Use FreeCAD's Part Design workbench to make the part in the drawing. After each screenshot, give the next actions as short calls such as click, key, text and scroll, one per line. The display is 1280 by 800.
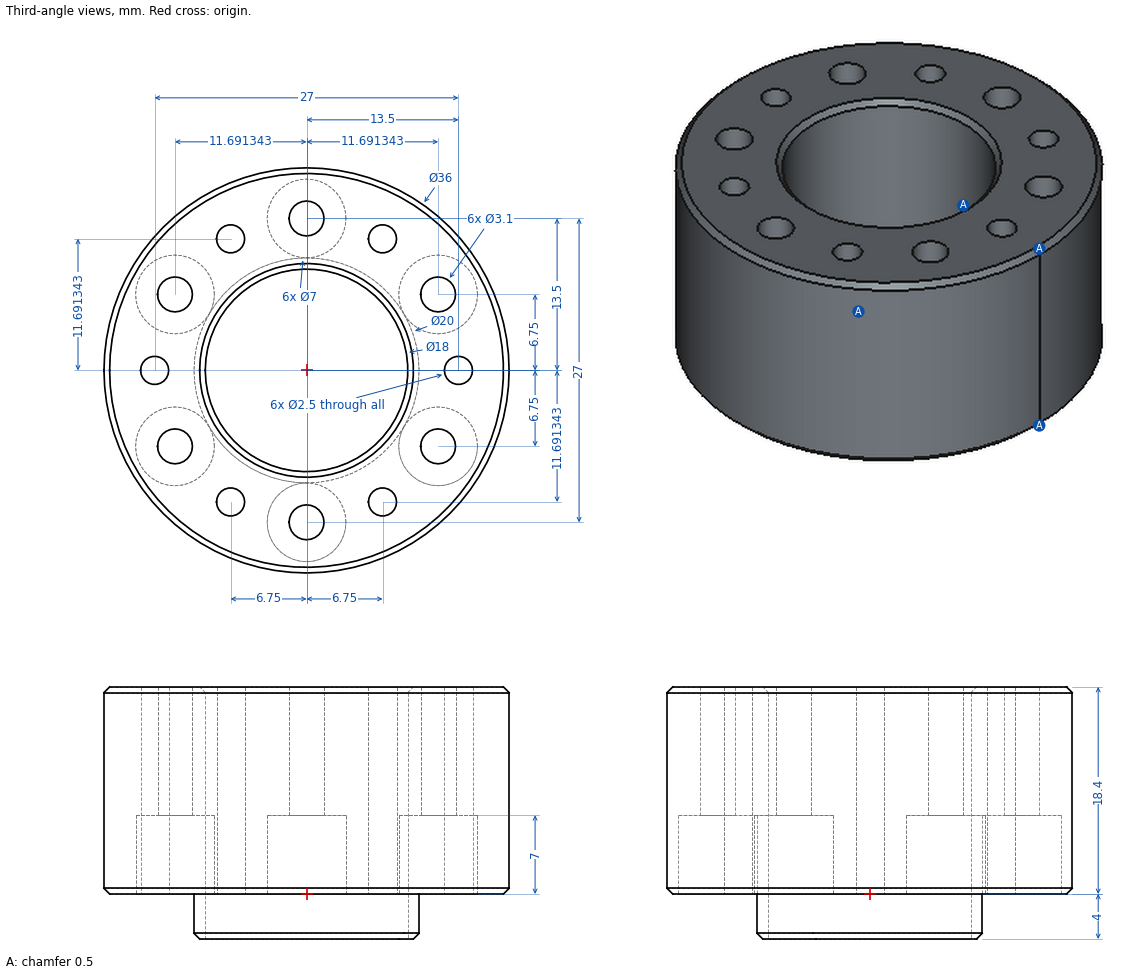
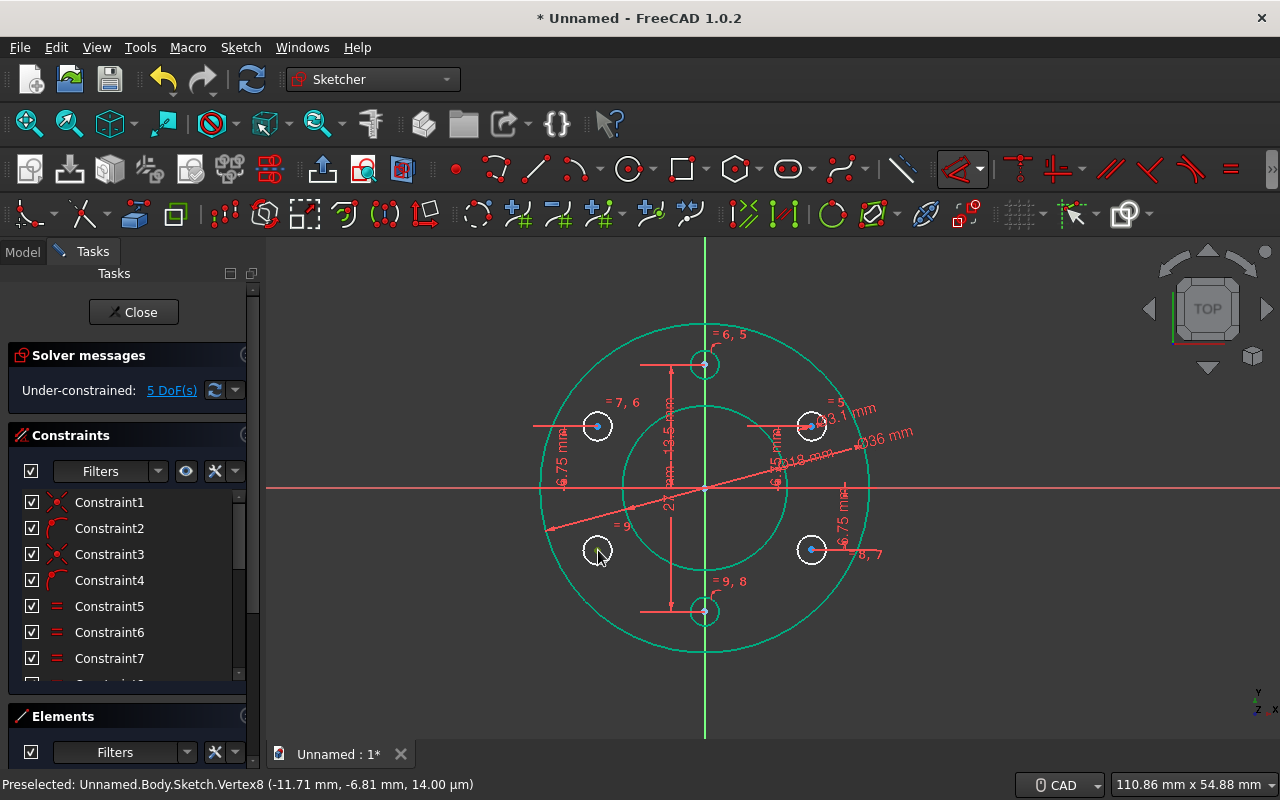
click(982, 170)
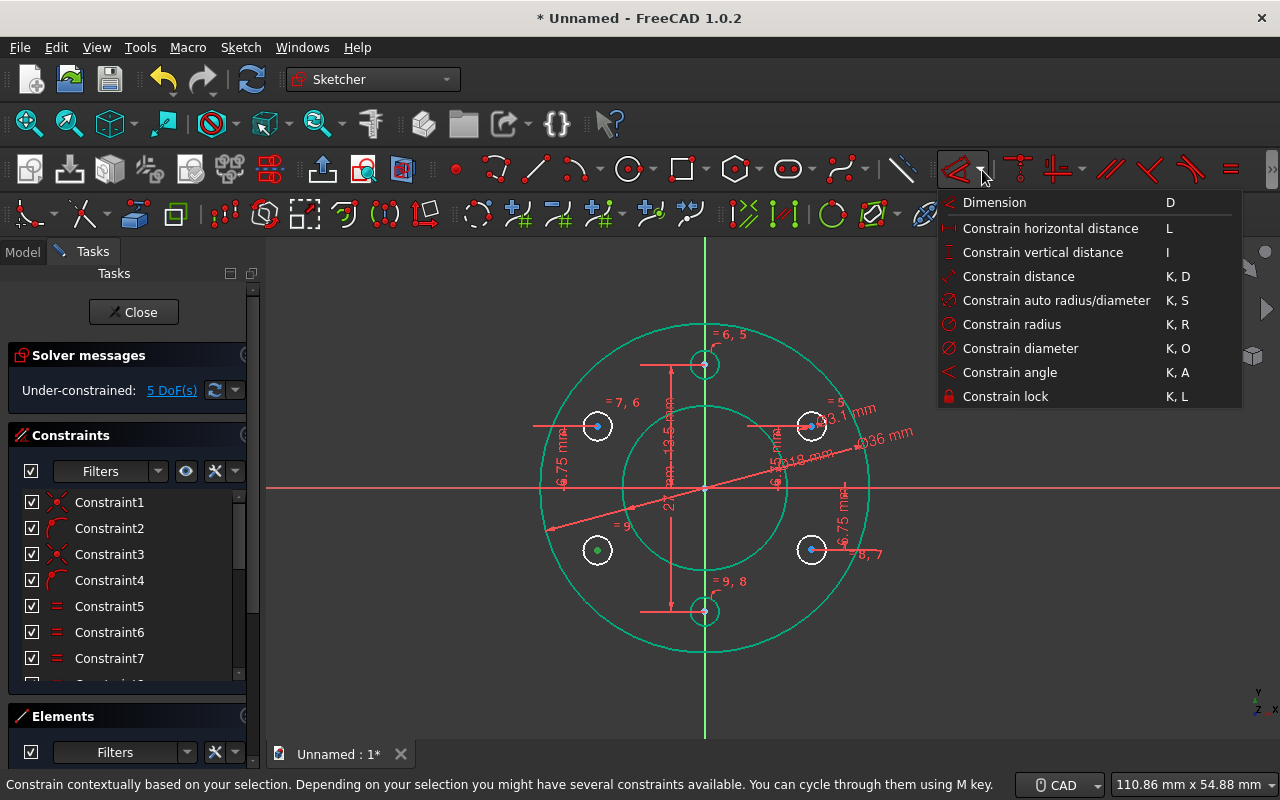
click(1090, 252)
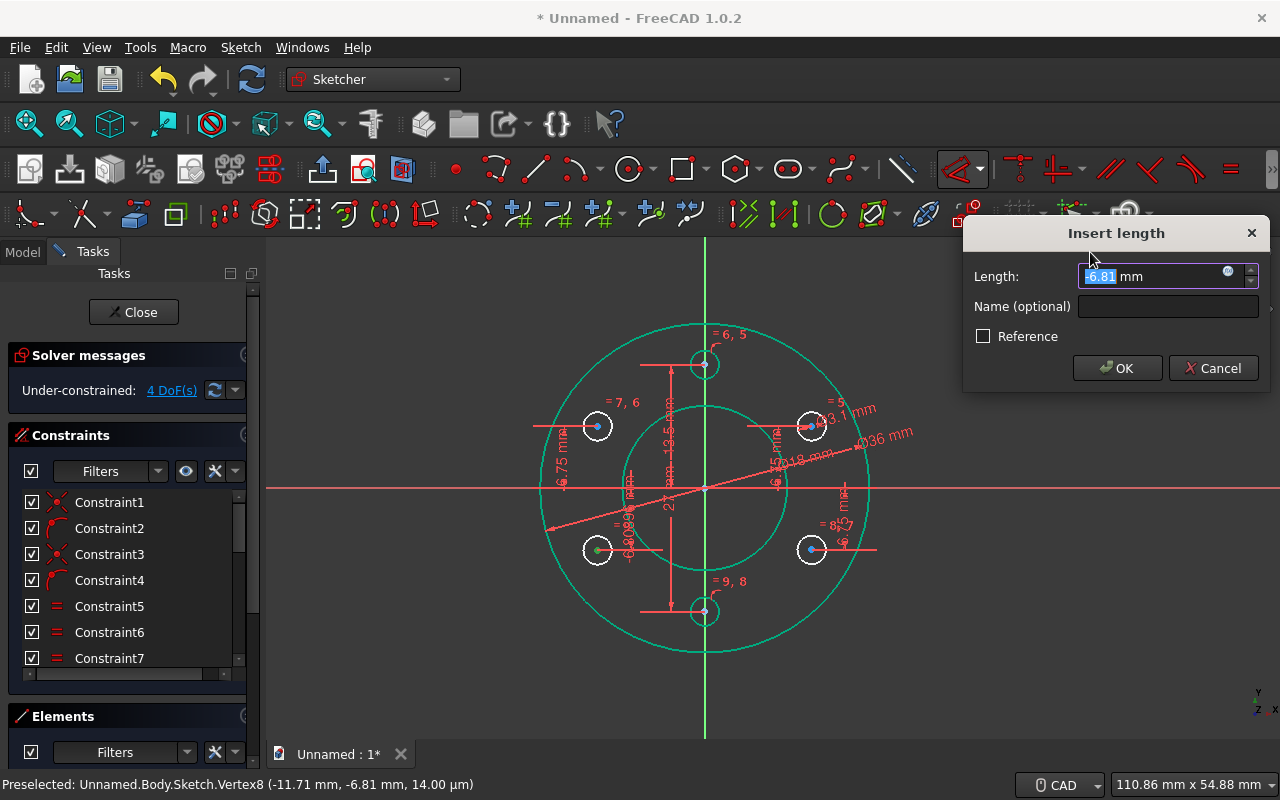
text(-6.75)
key(Return)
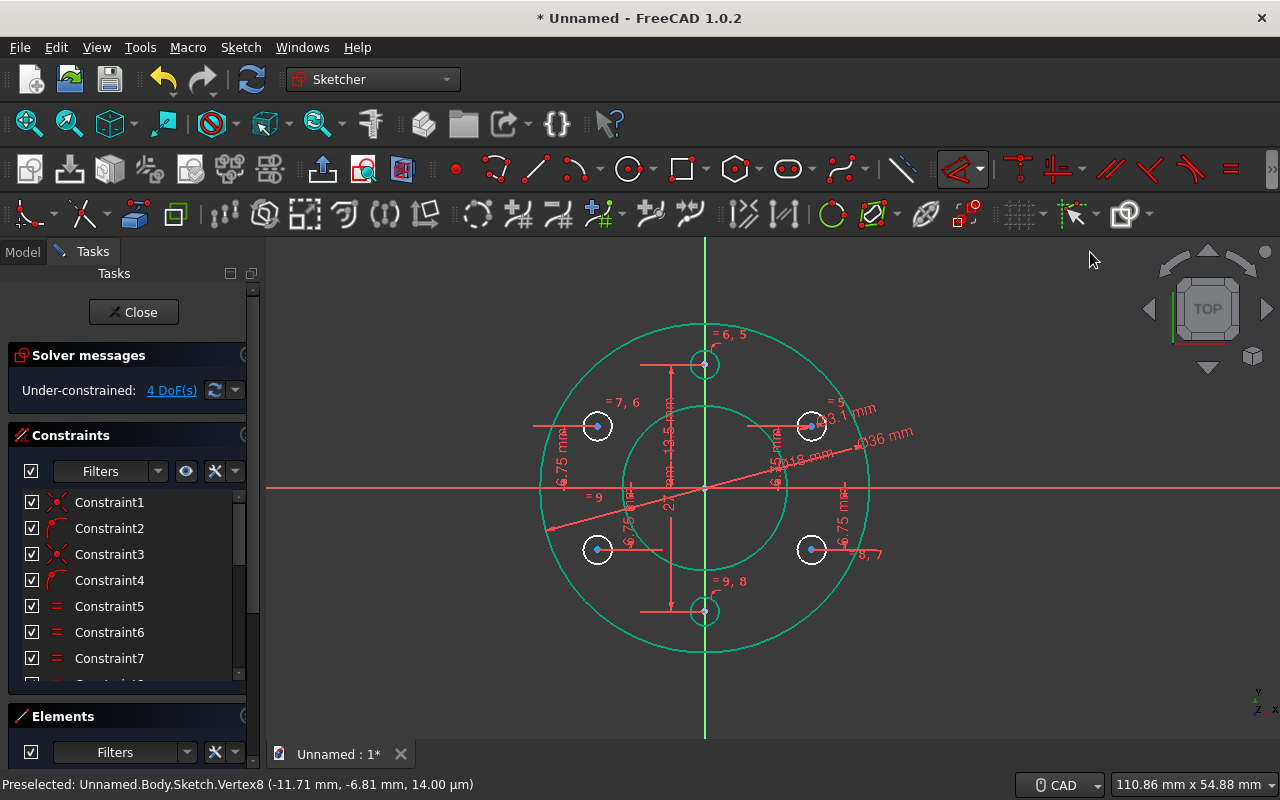
click(812, 426)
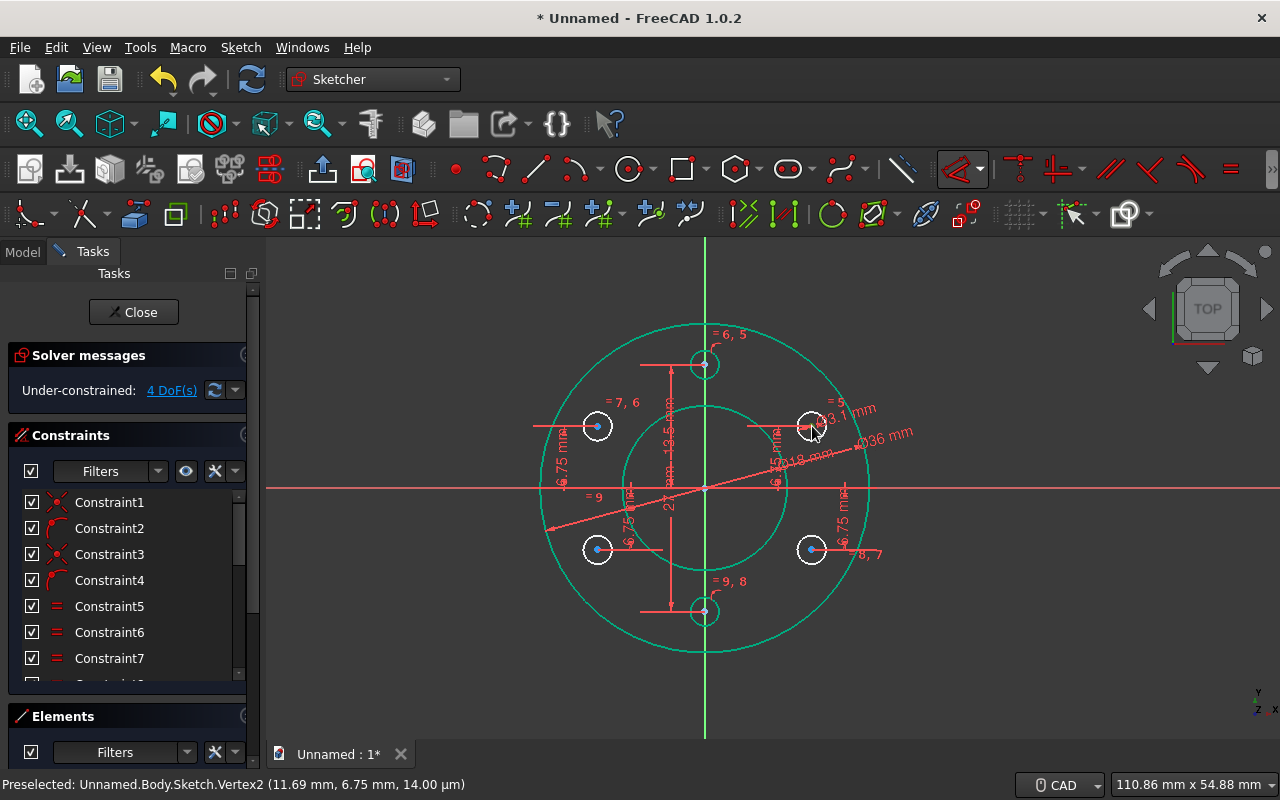
key(l)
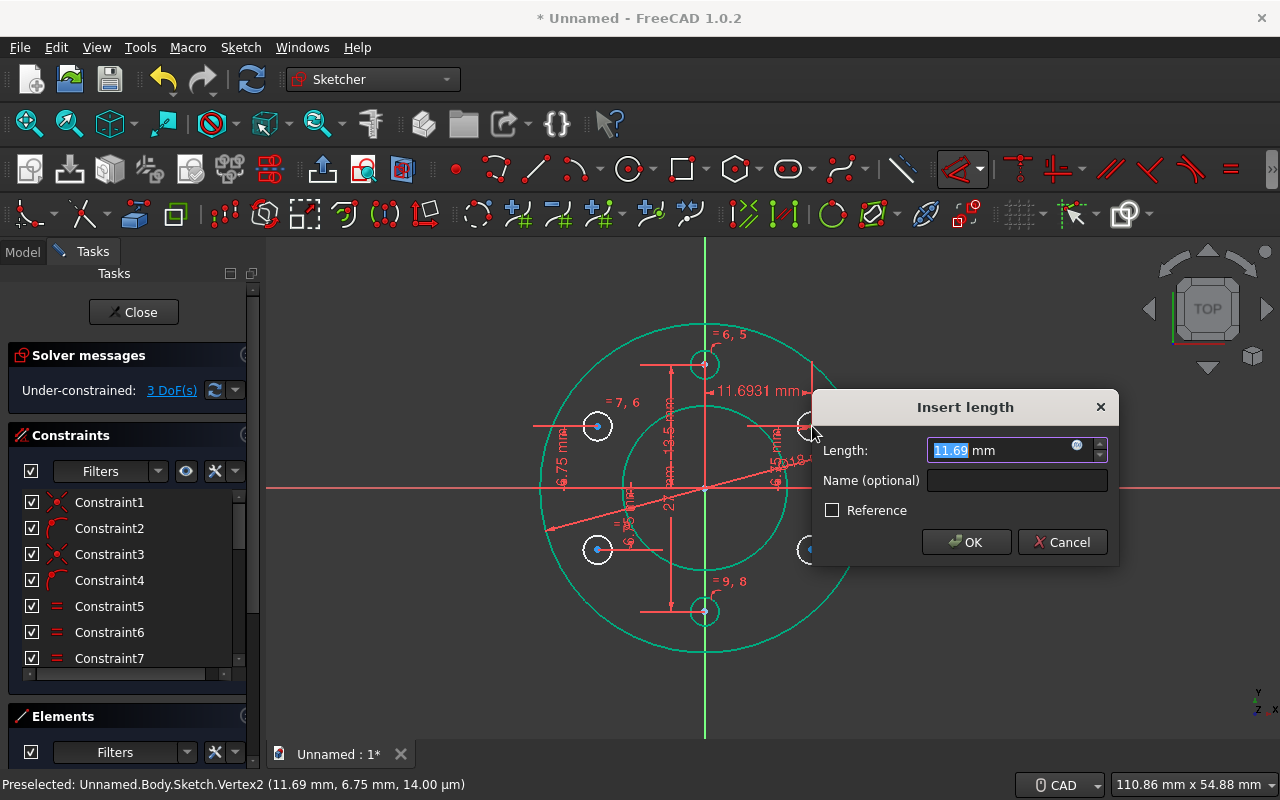
text(11.691343)
key(Return)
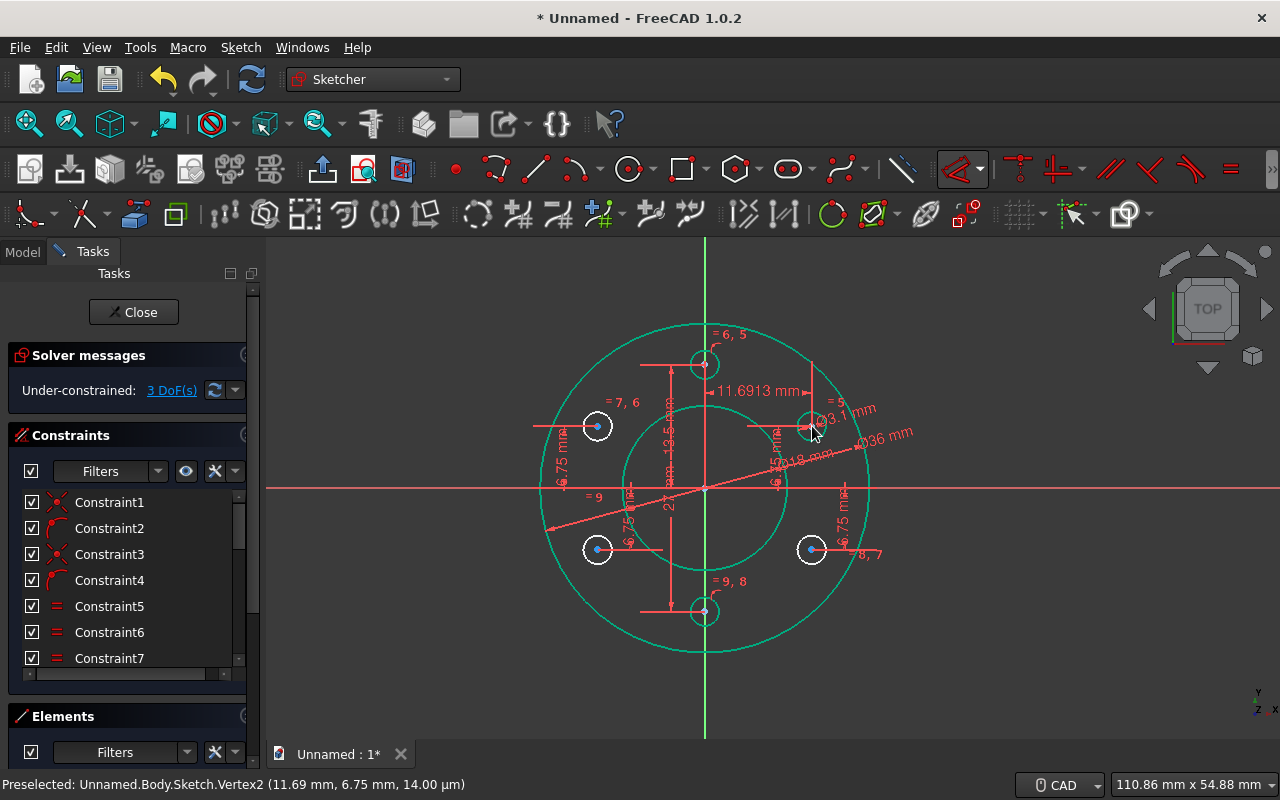
click(598, 426)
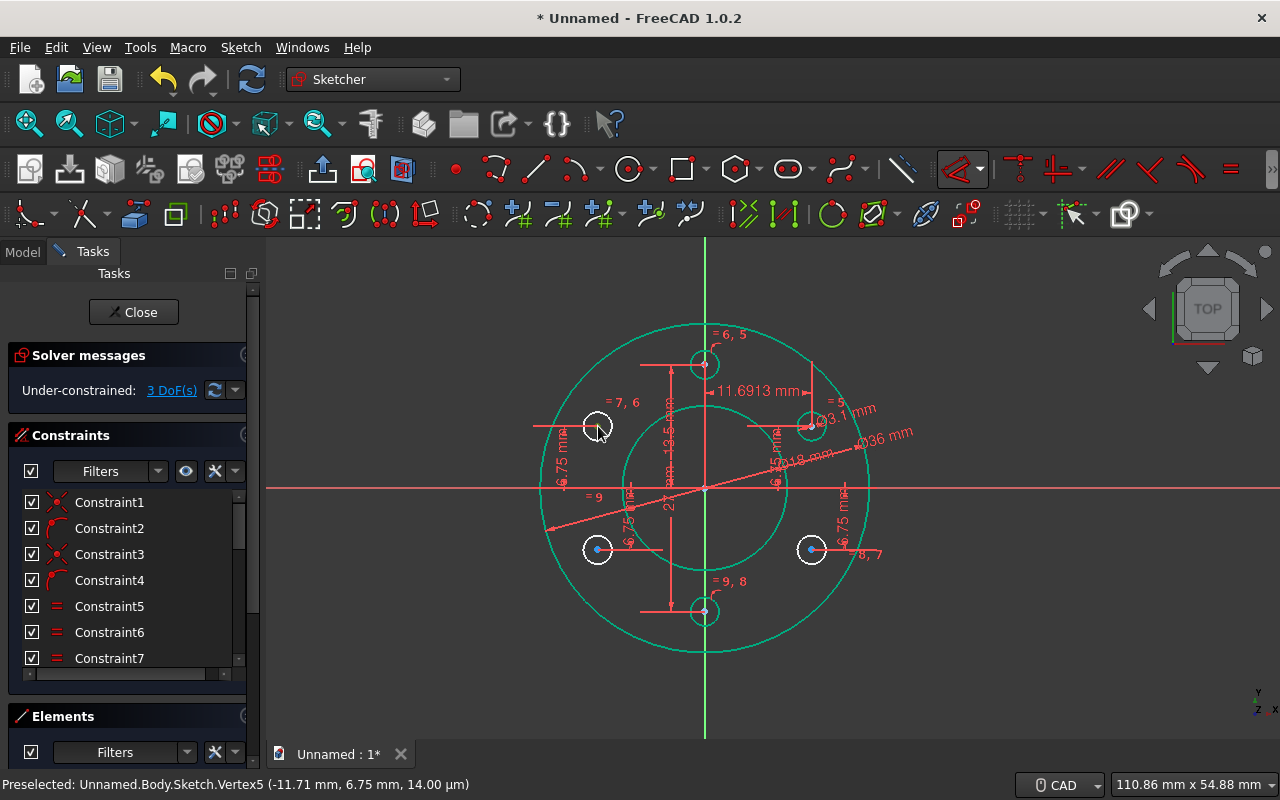
click(982, 170)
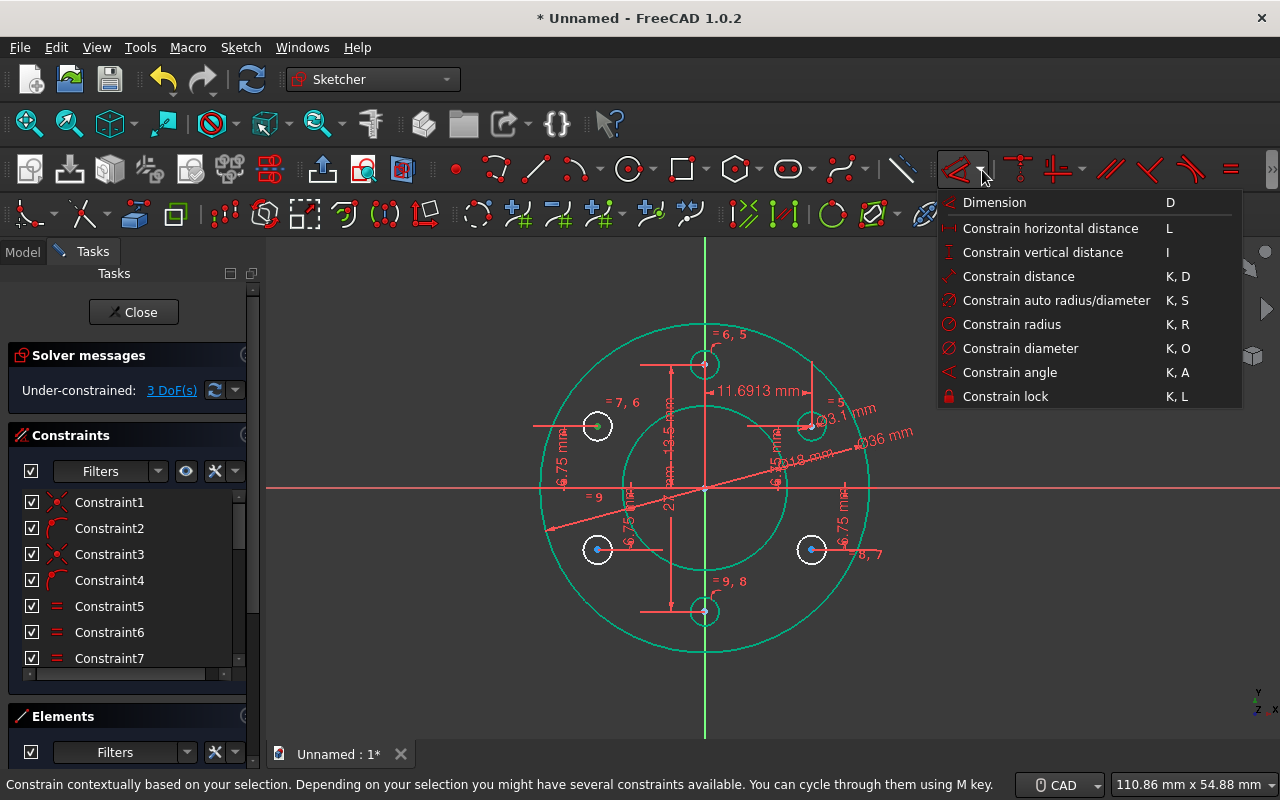
click(1090, 228)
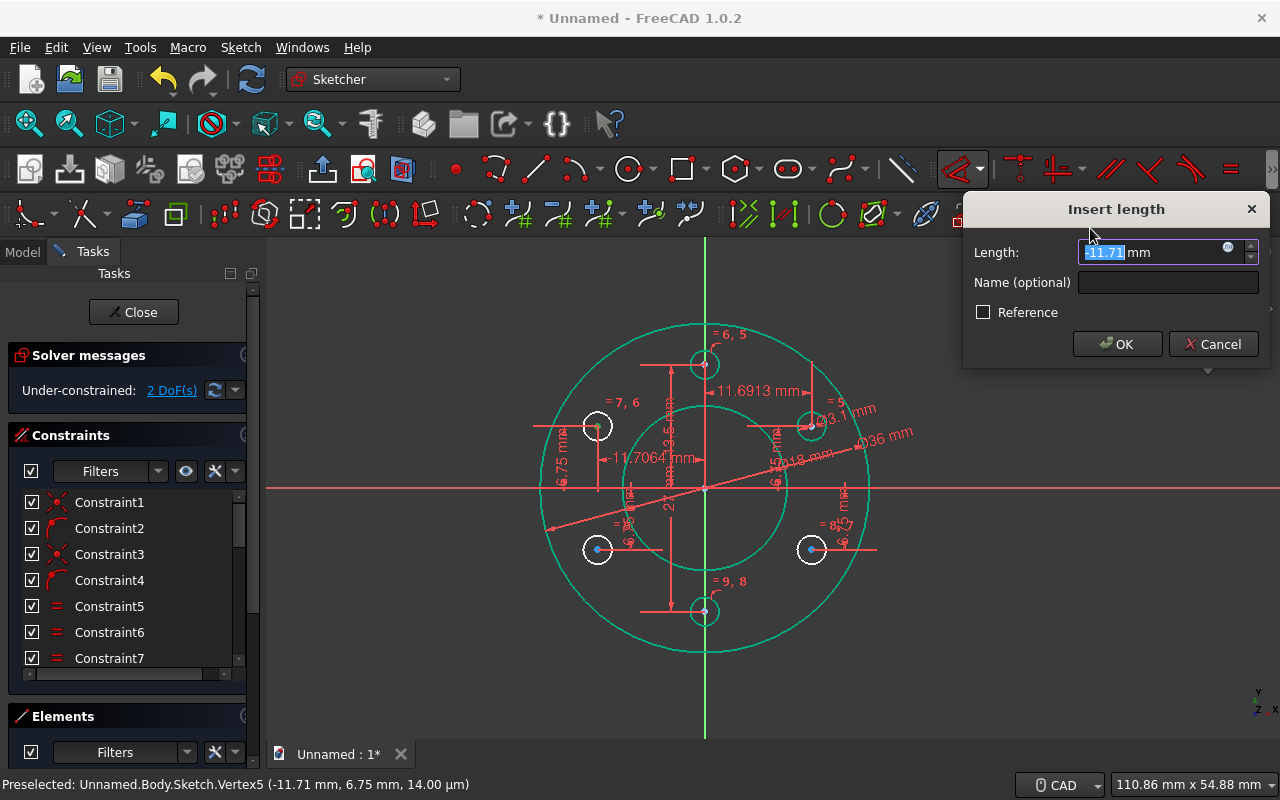
text(-11.691343)
key(Return)